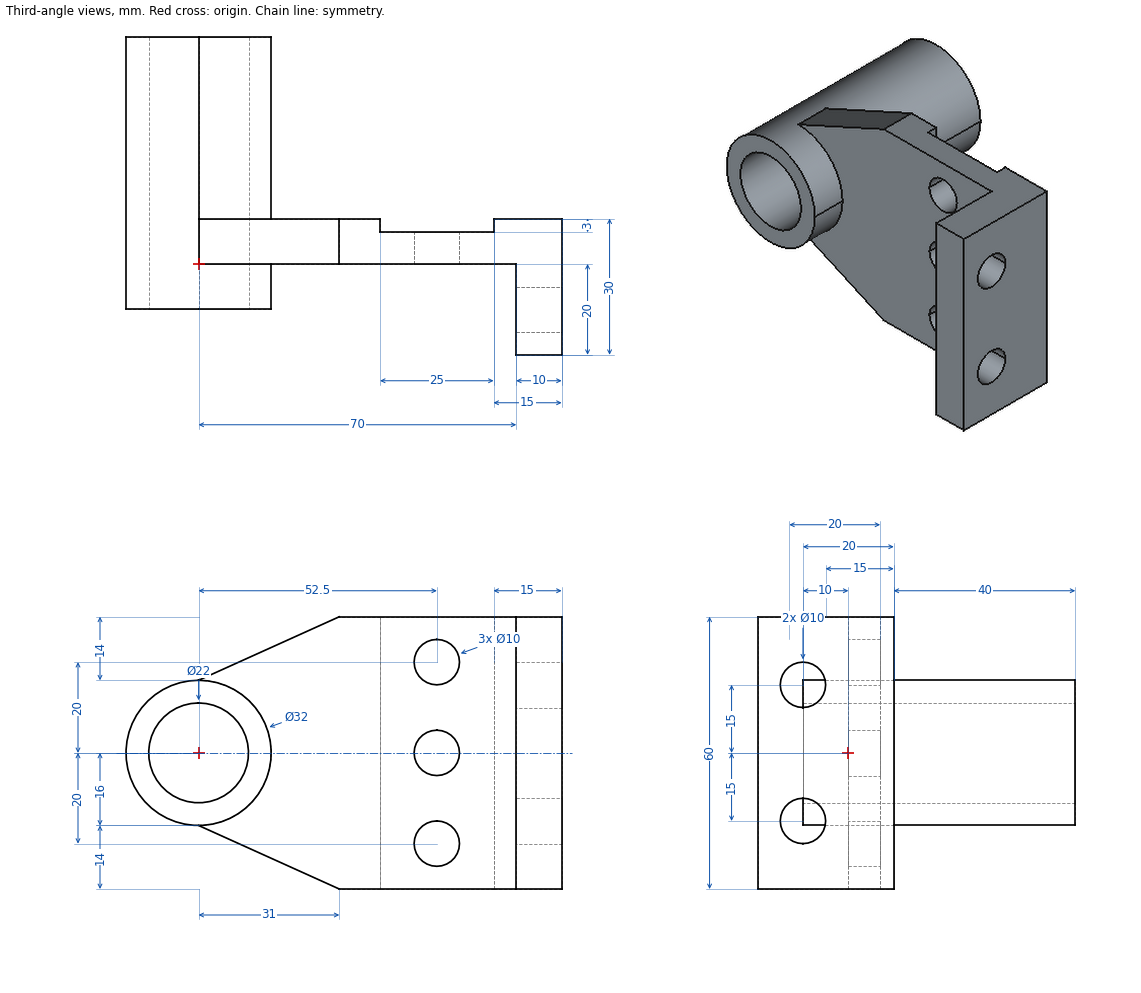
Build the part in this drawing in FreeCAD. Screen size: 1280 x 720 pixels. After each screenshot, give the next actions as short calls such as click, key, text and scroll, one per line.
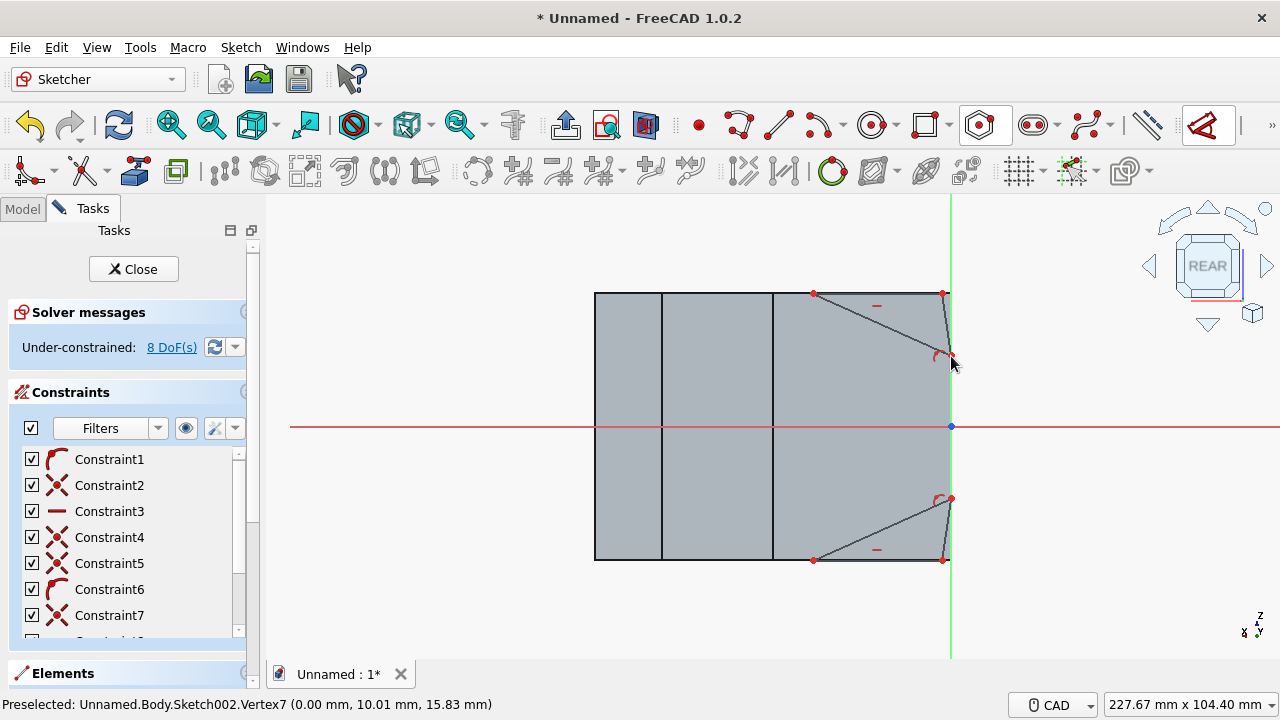
click(948, 518)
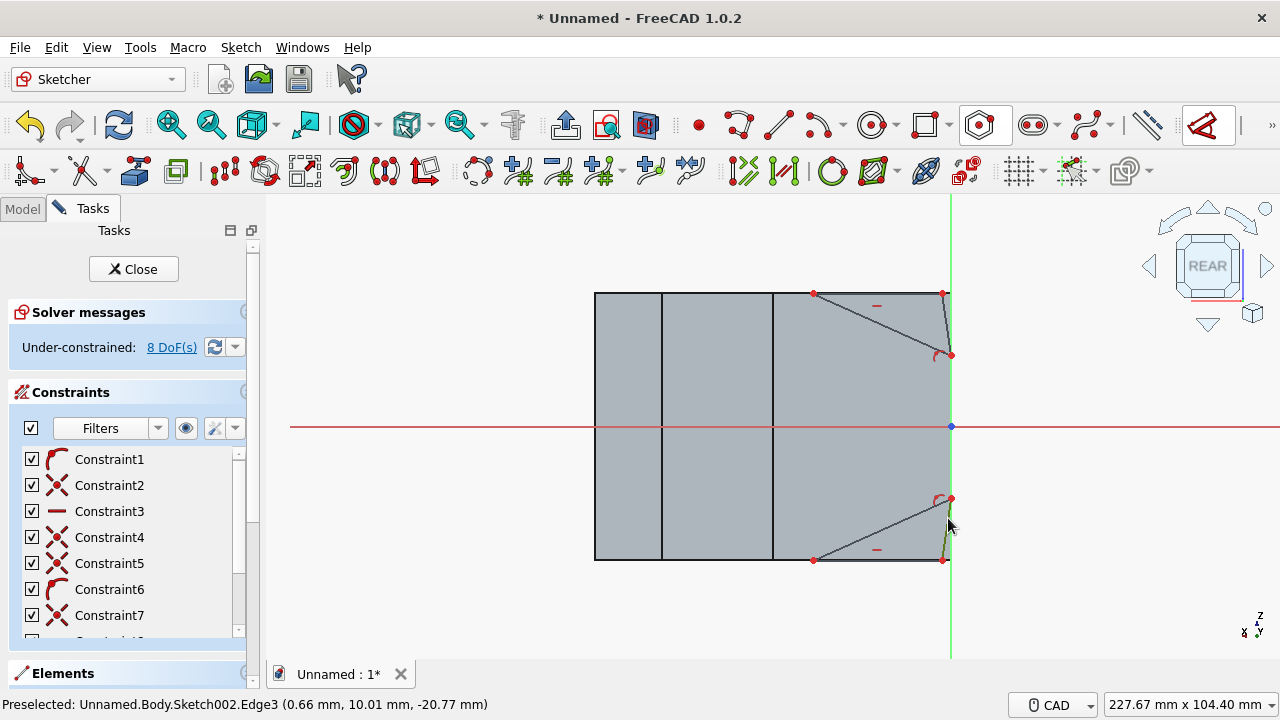
key(v)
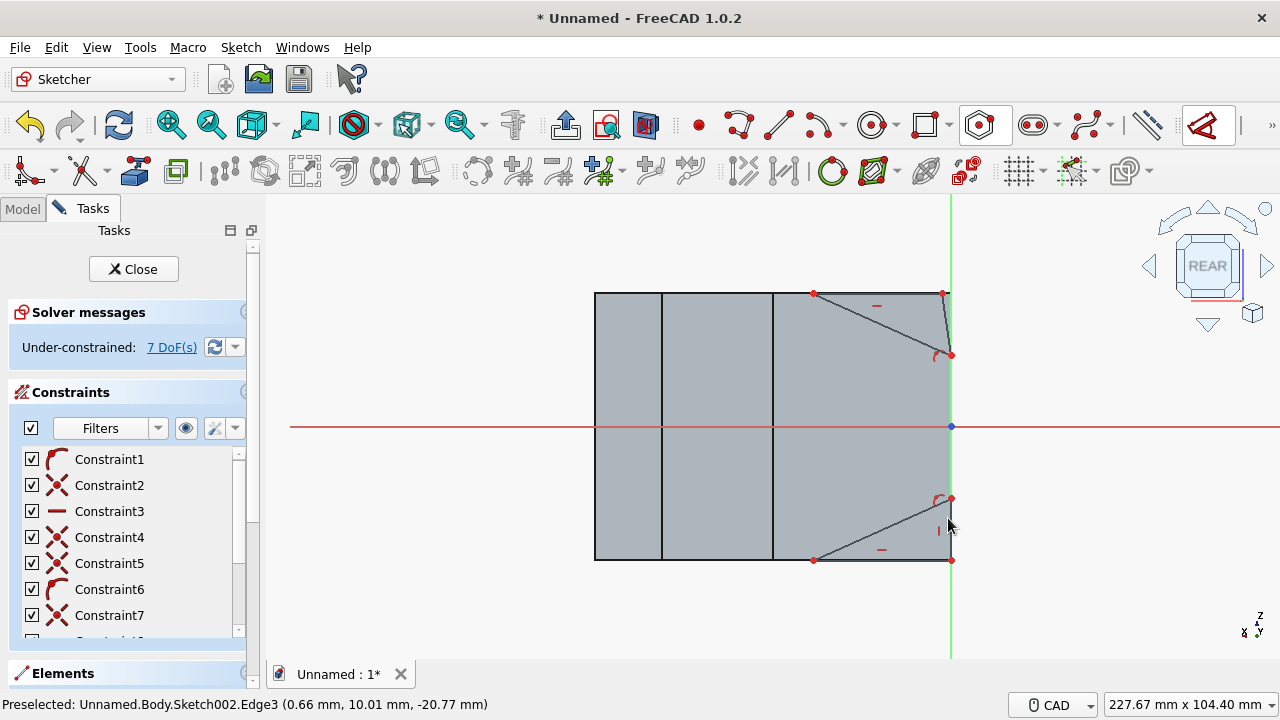
click(948, 337)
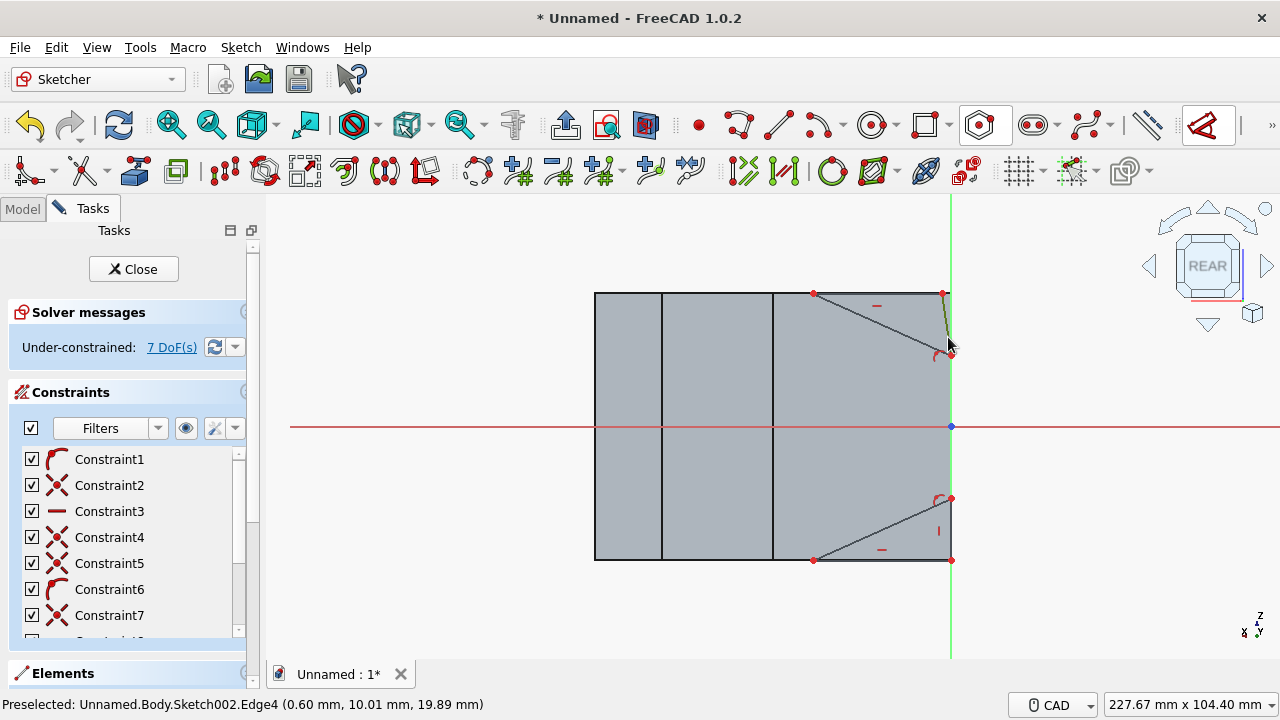
key(v)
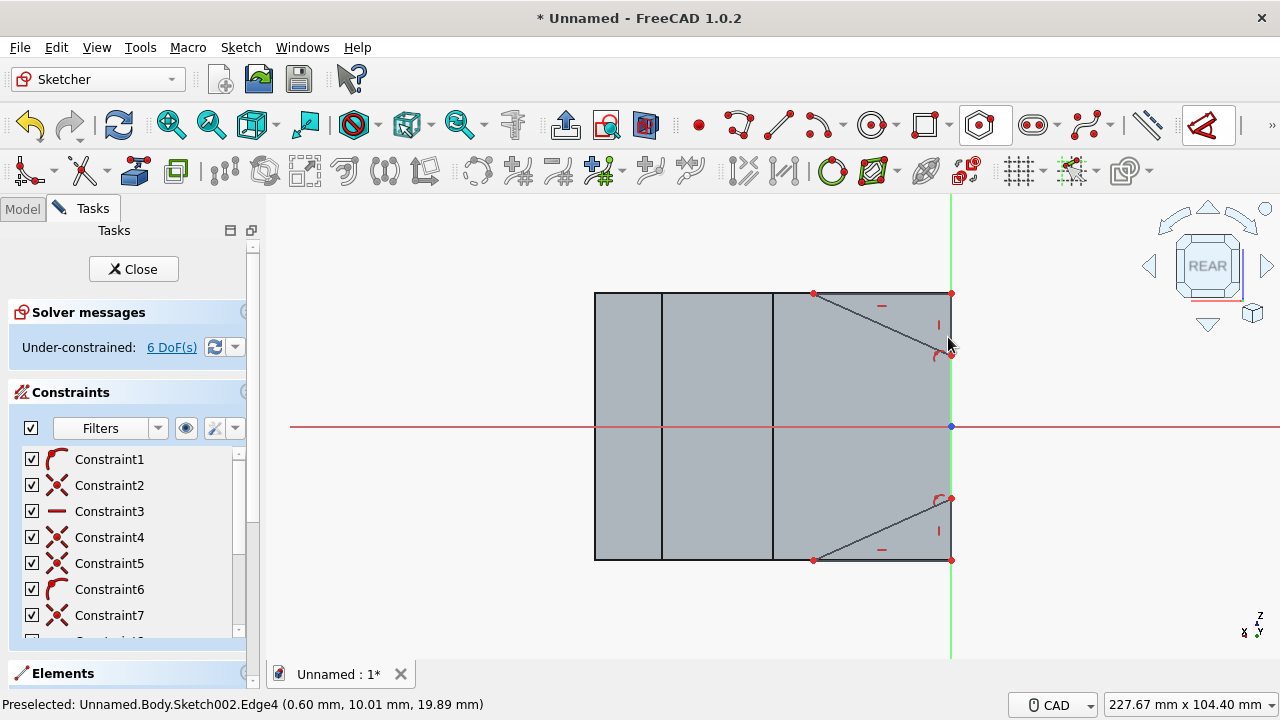
click(813, 561)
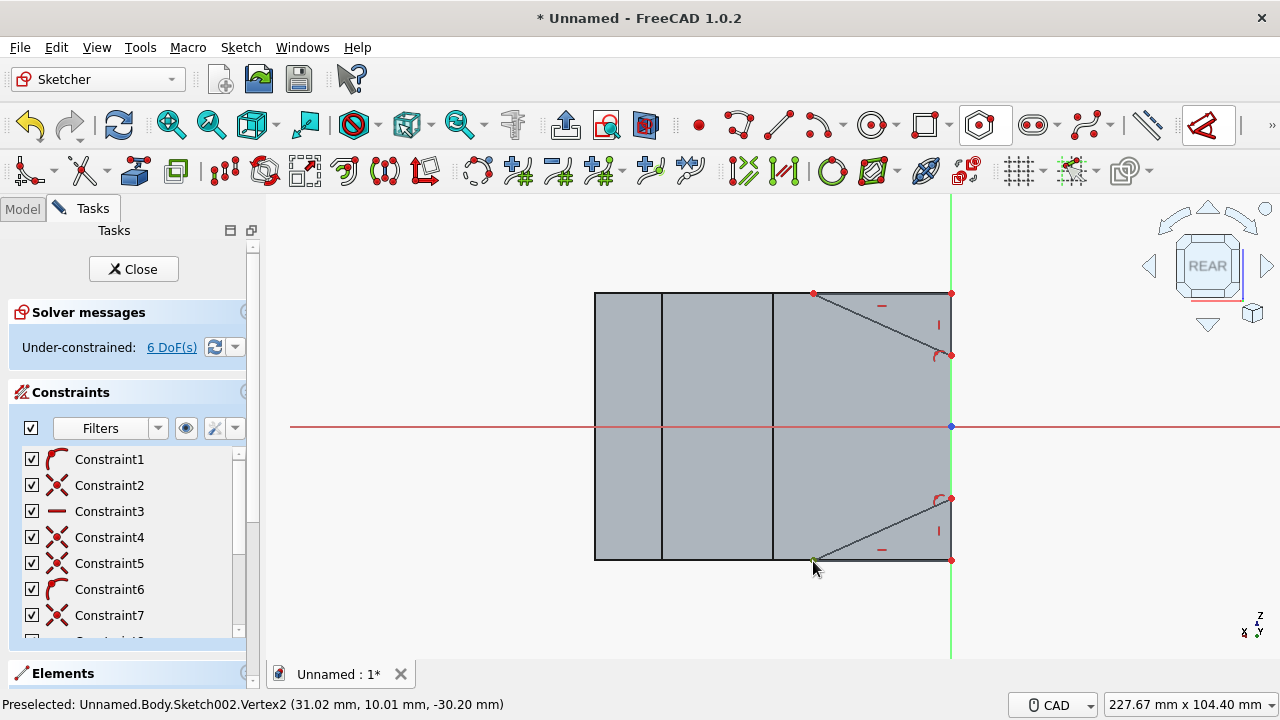
click(813, 294)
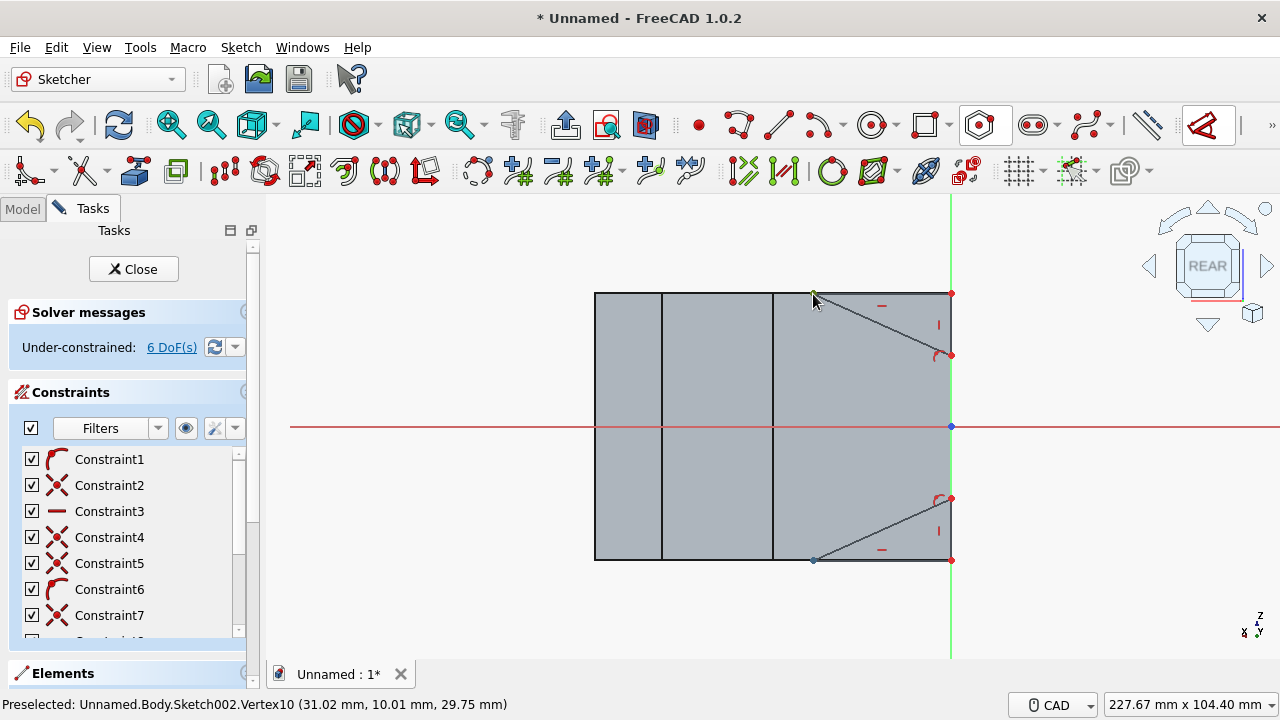
click(353, 426)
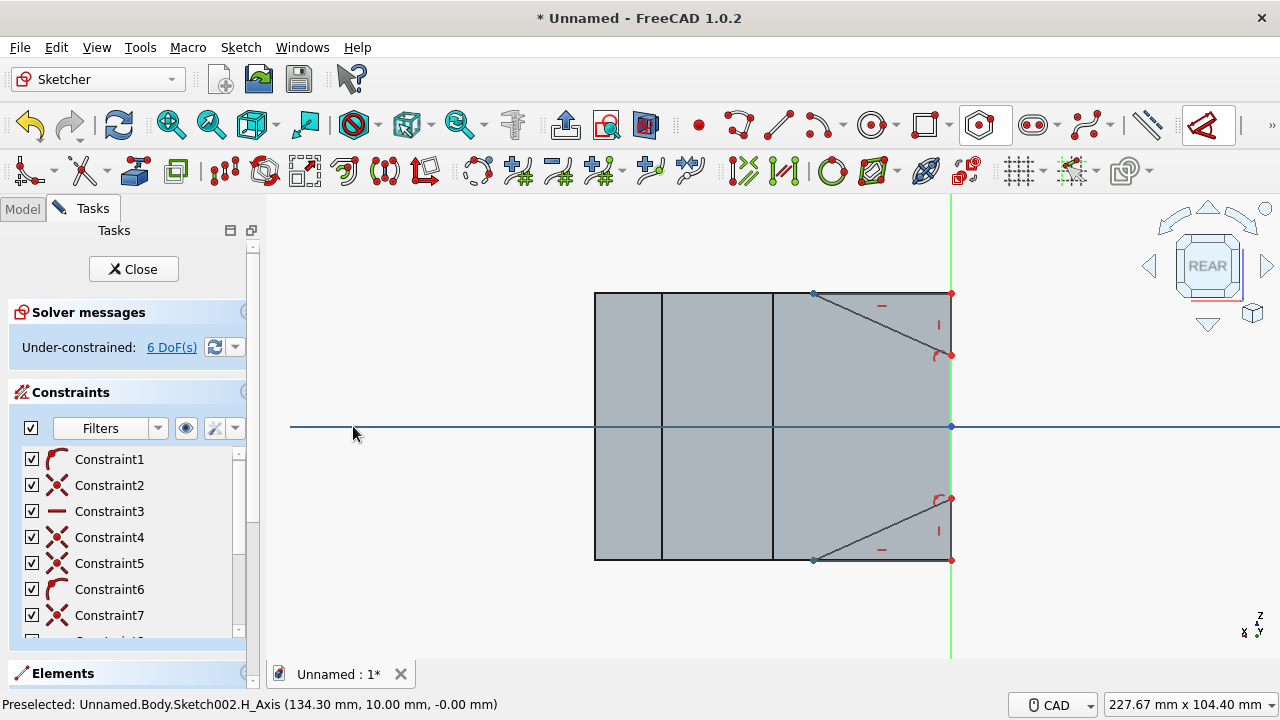
key(s)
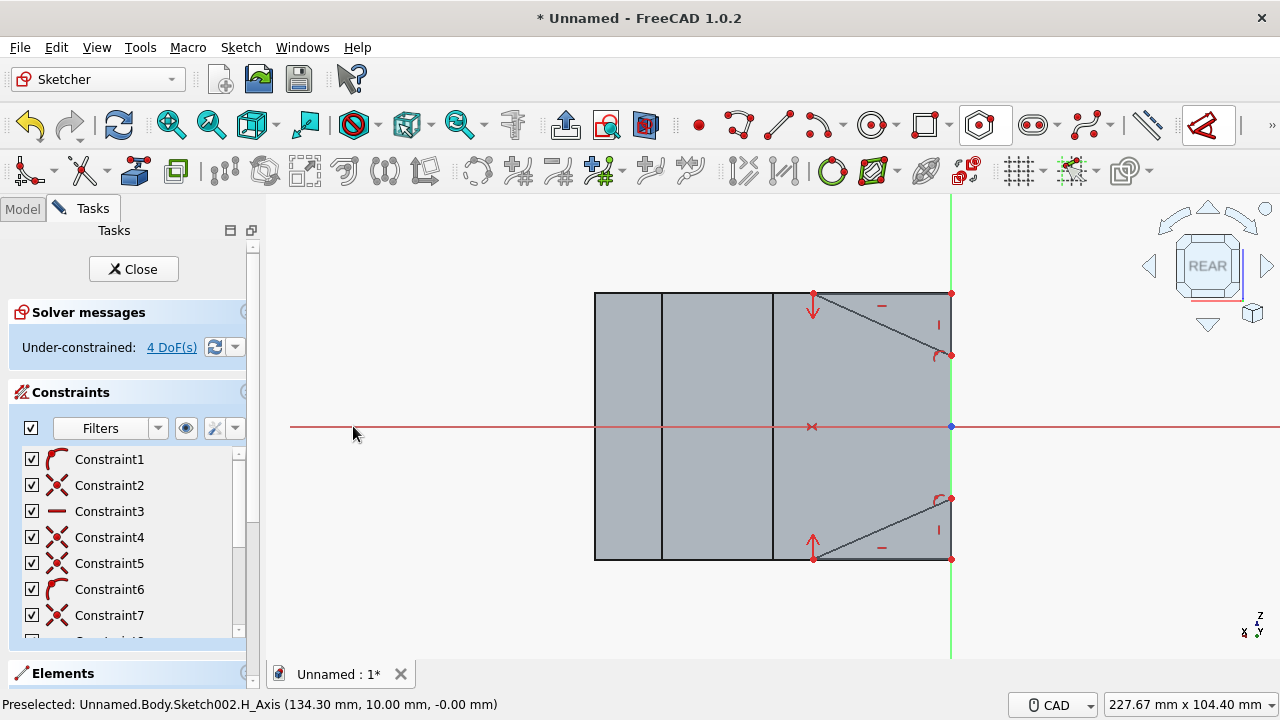
click(854, 559)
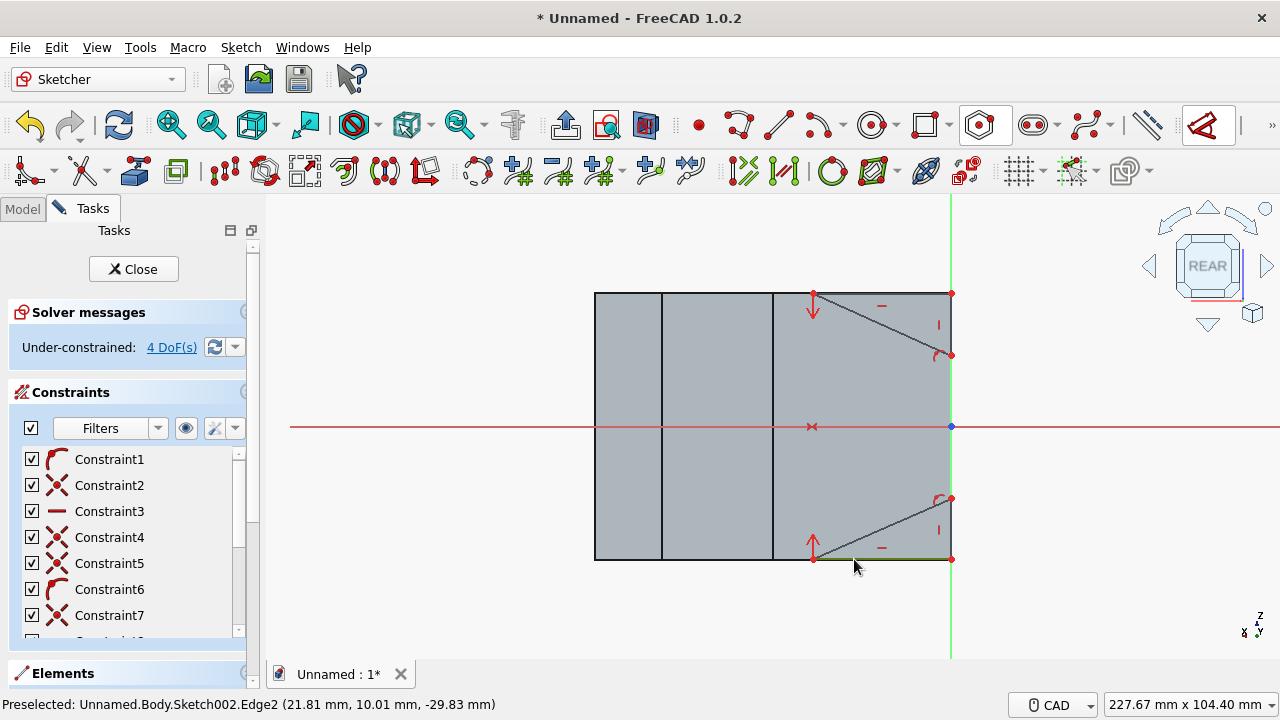
key(l)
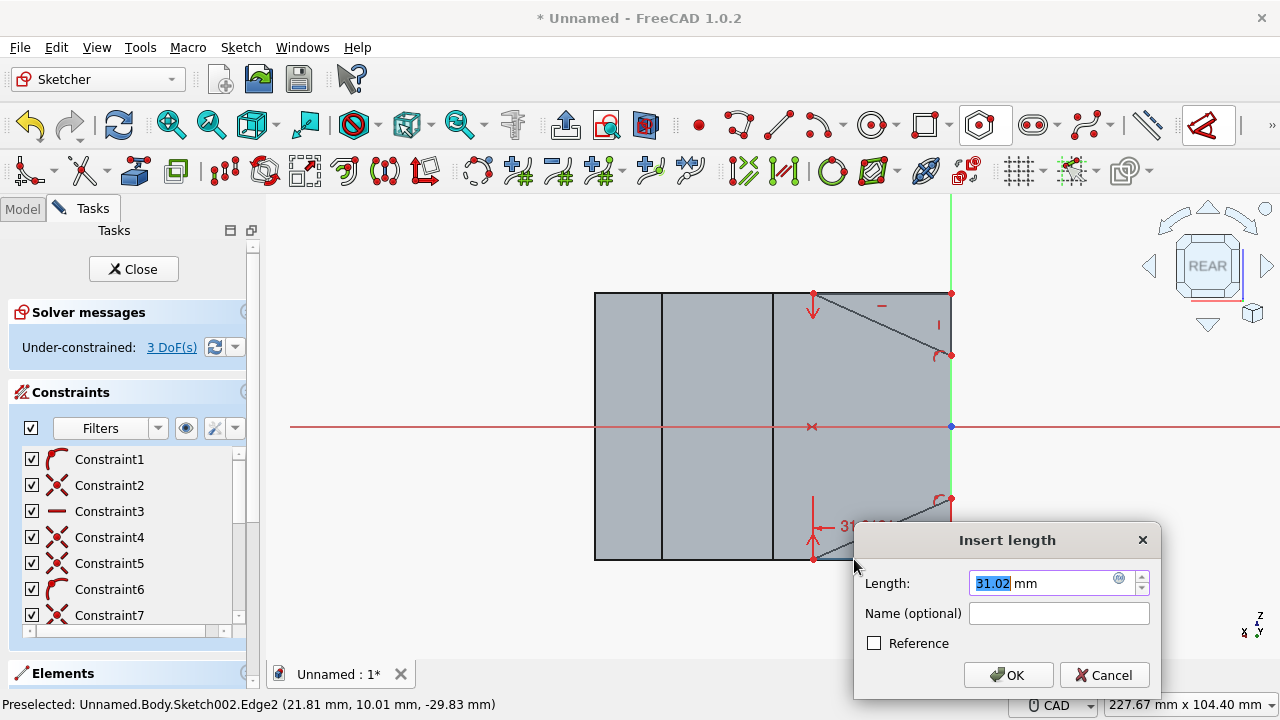
text(31)
key(Return)